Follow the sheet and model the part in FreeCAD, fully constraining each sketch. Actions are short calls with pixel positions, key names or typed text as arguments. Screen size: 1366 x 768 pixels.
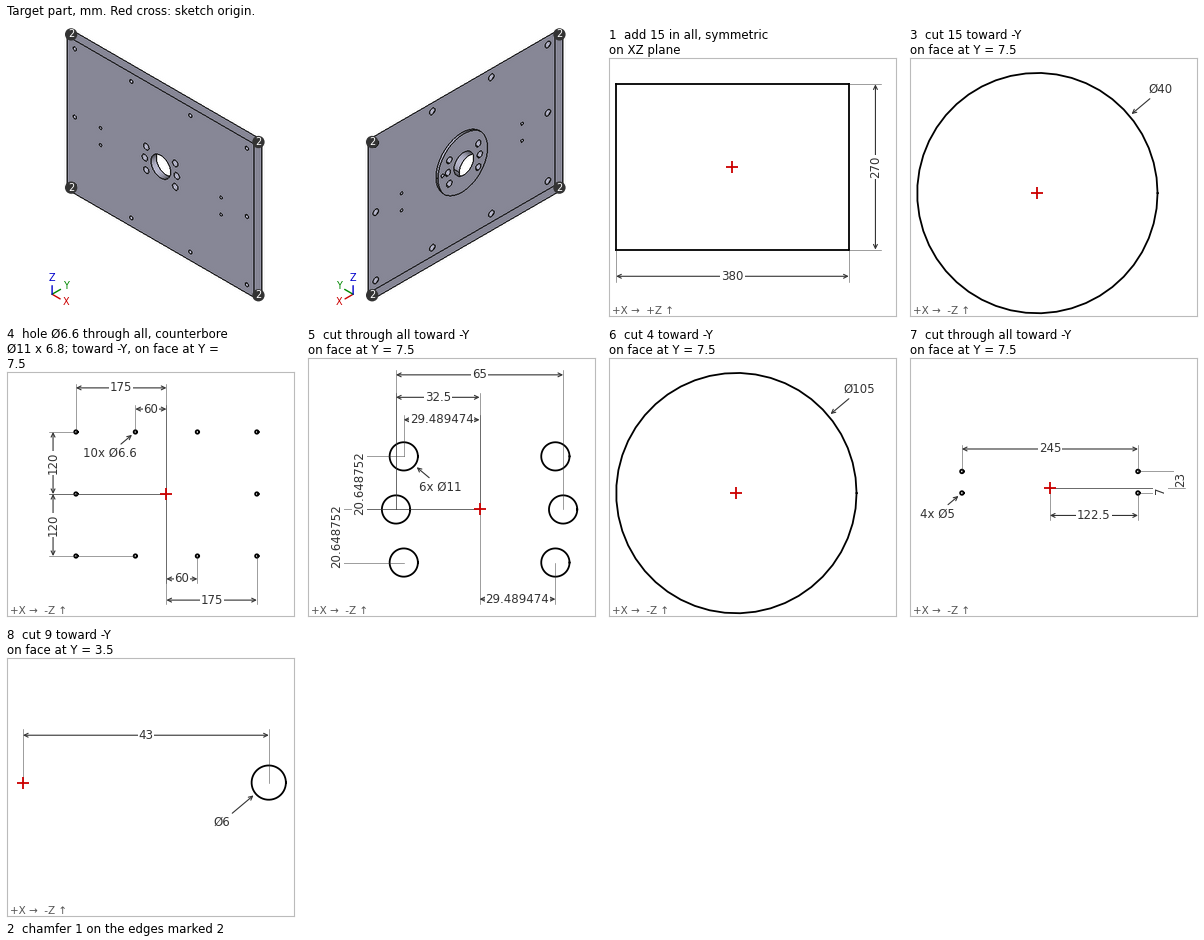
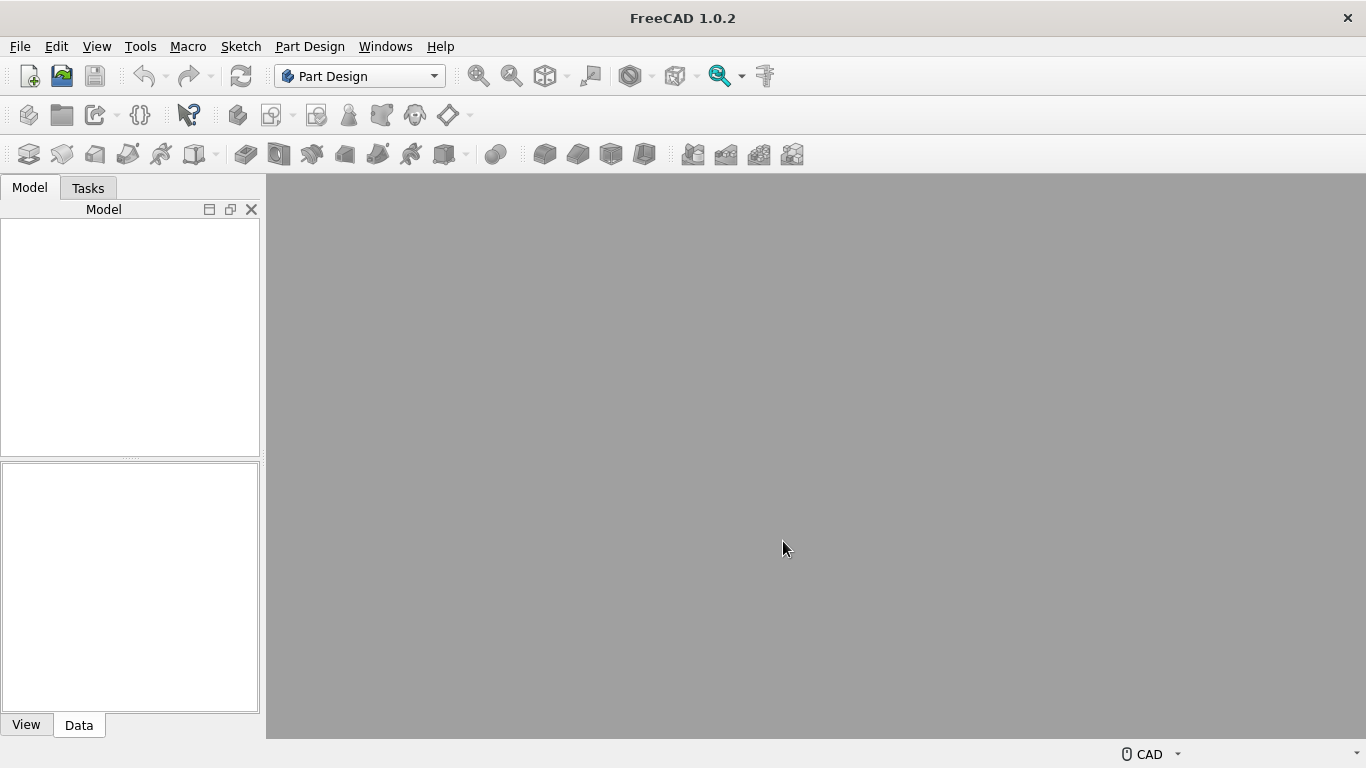
click(29, 76)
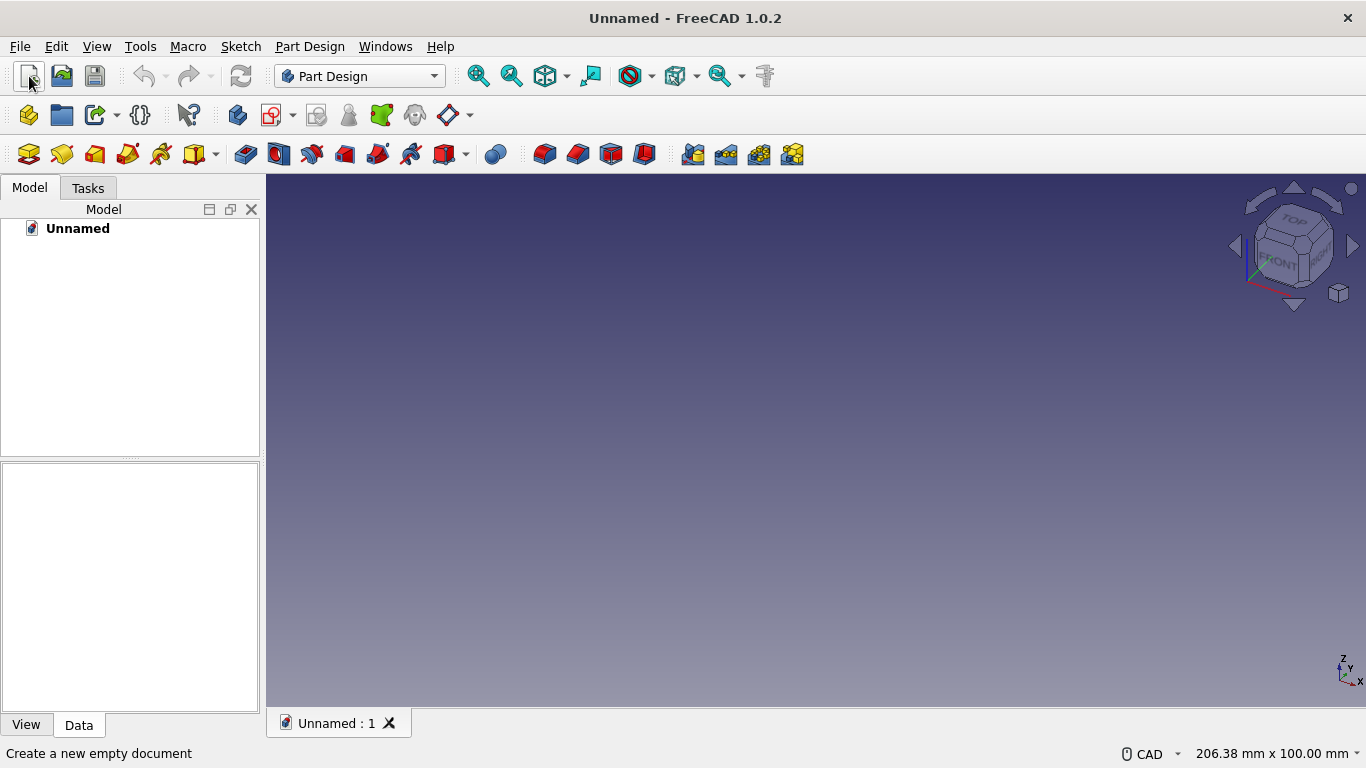
click(270, 116)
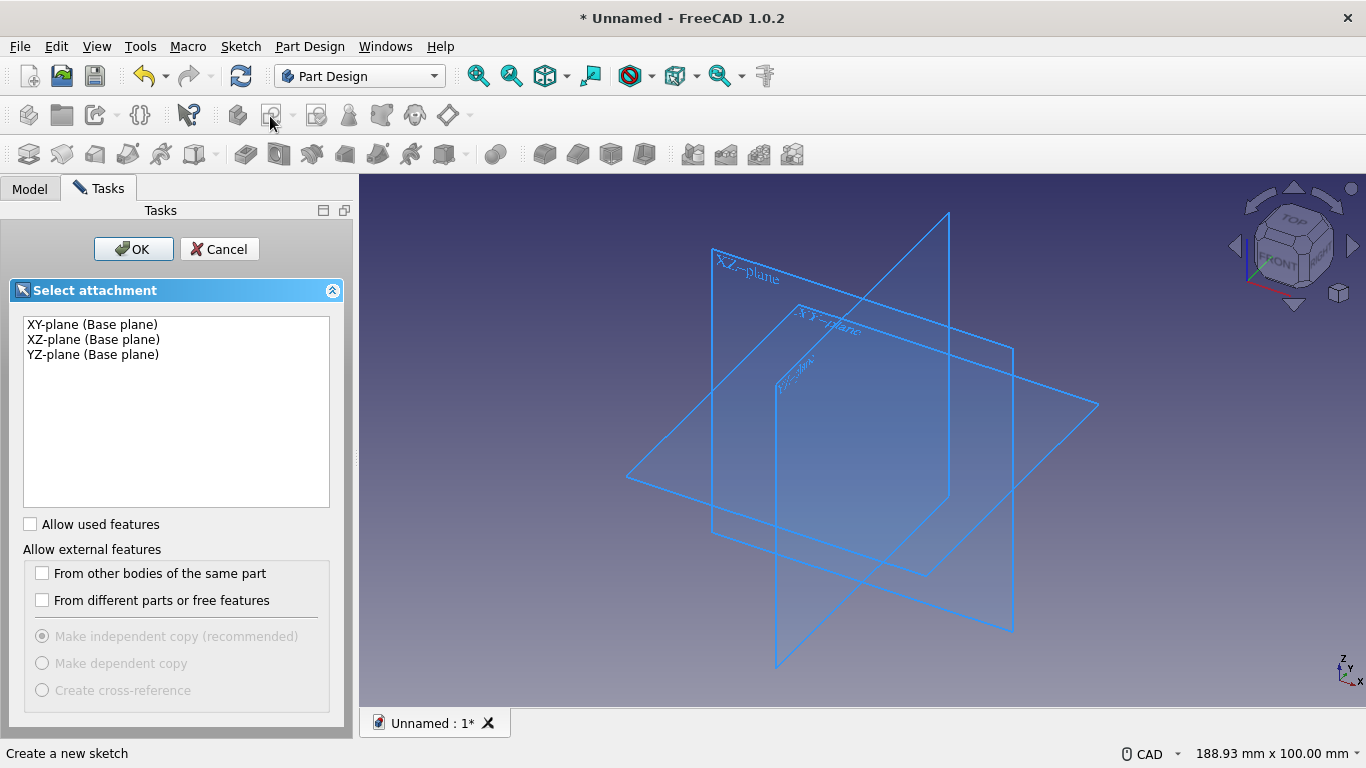
click(84, 340)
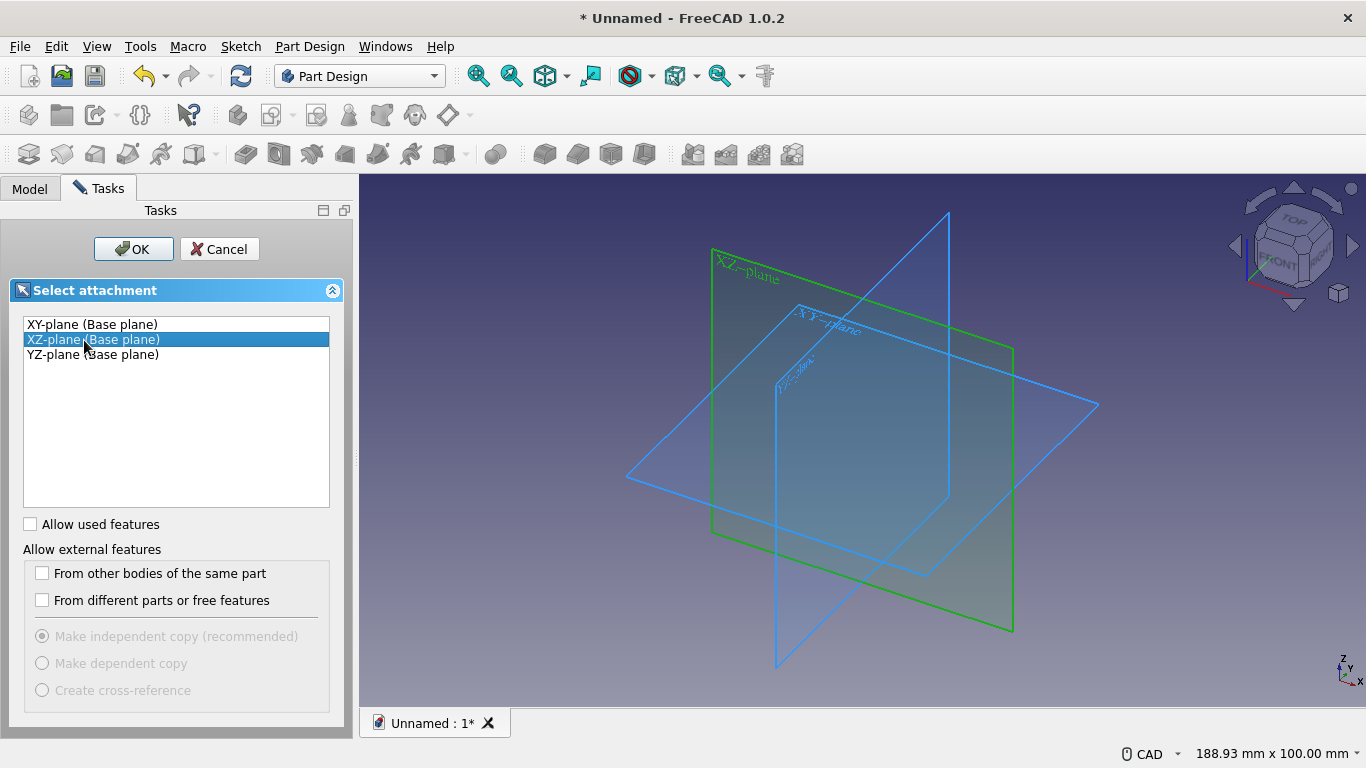
click(134, 249)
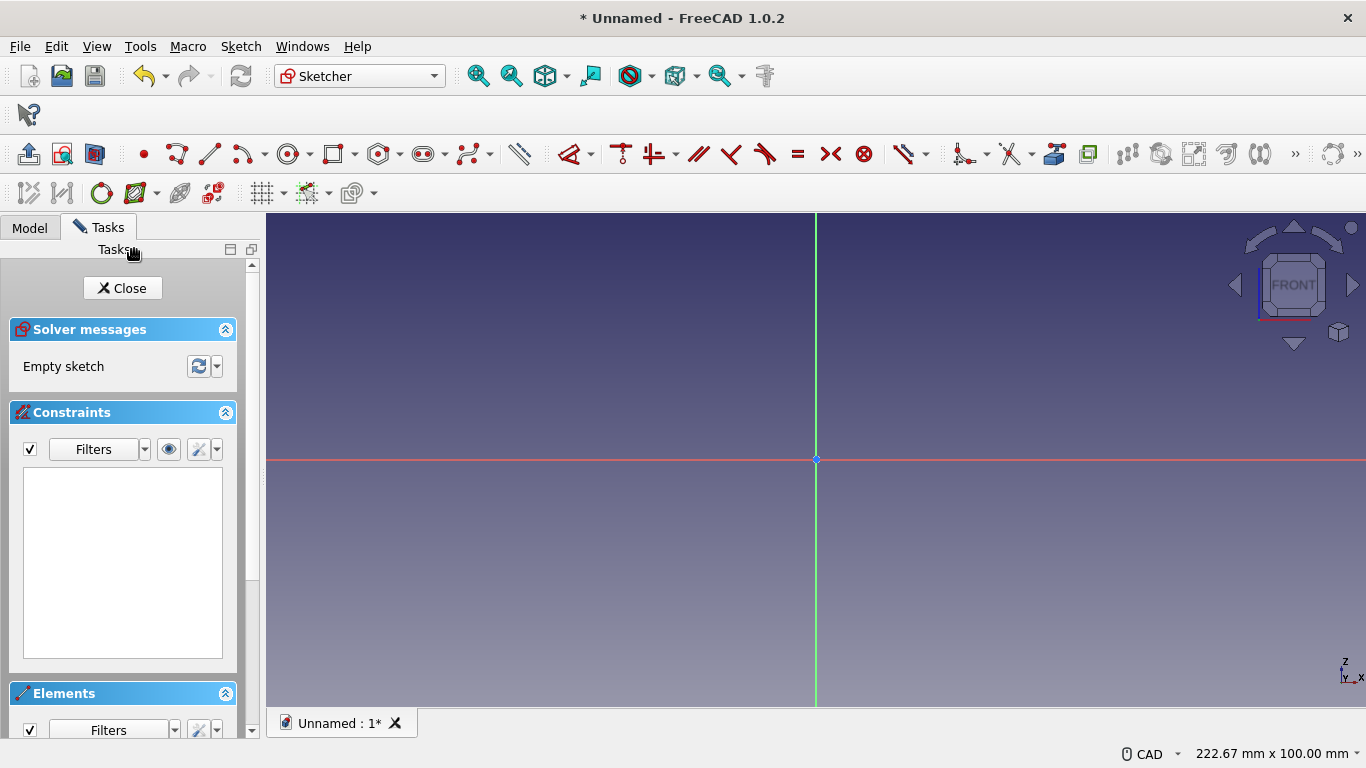
scroll(725, 460, down, 7)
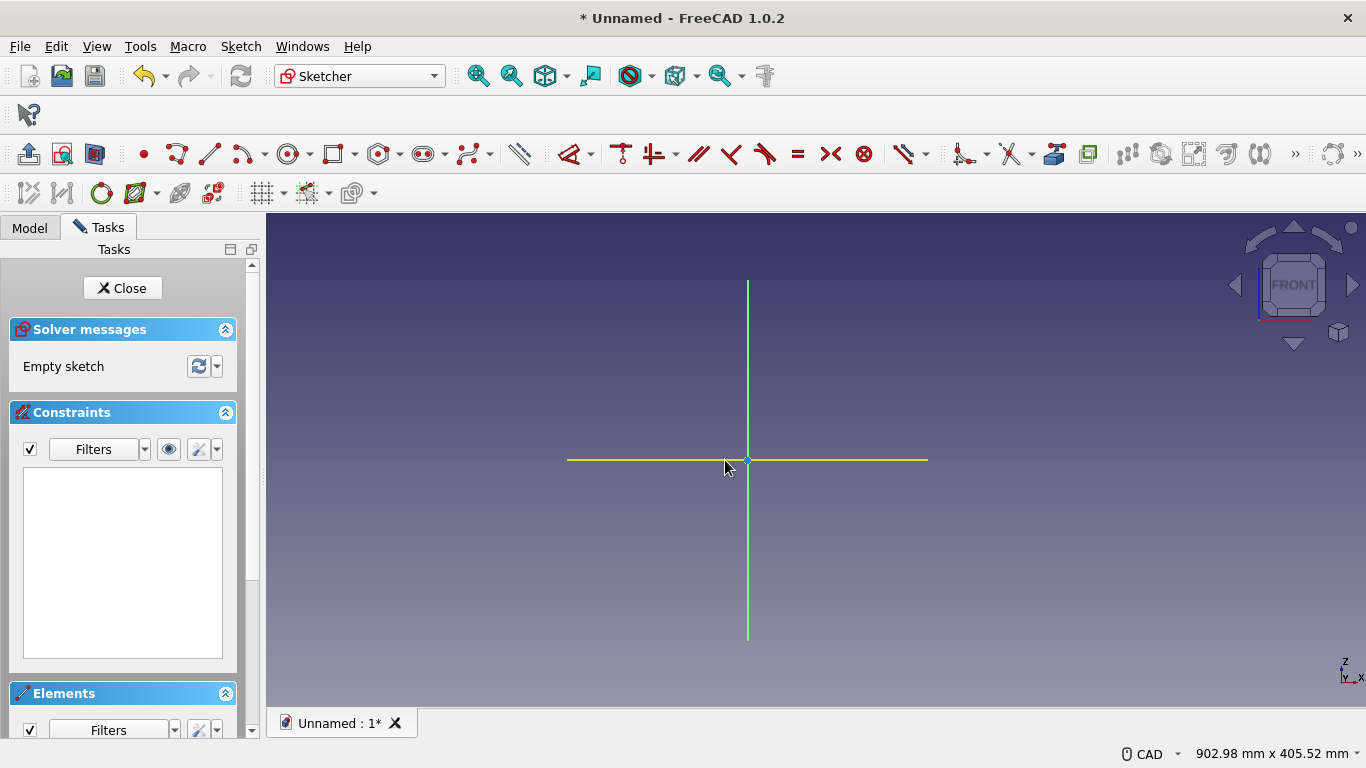
click(354, 154)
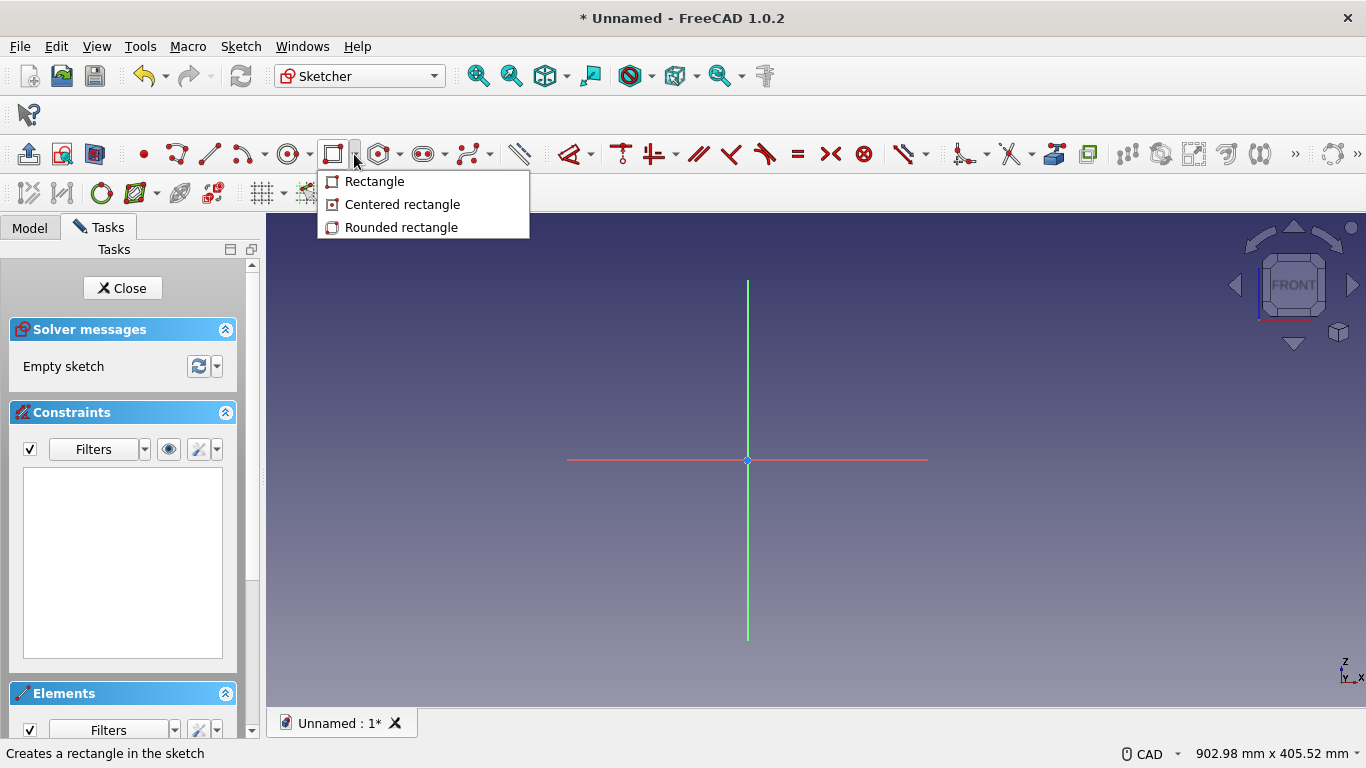
click(424, 204)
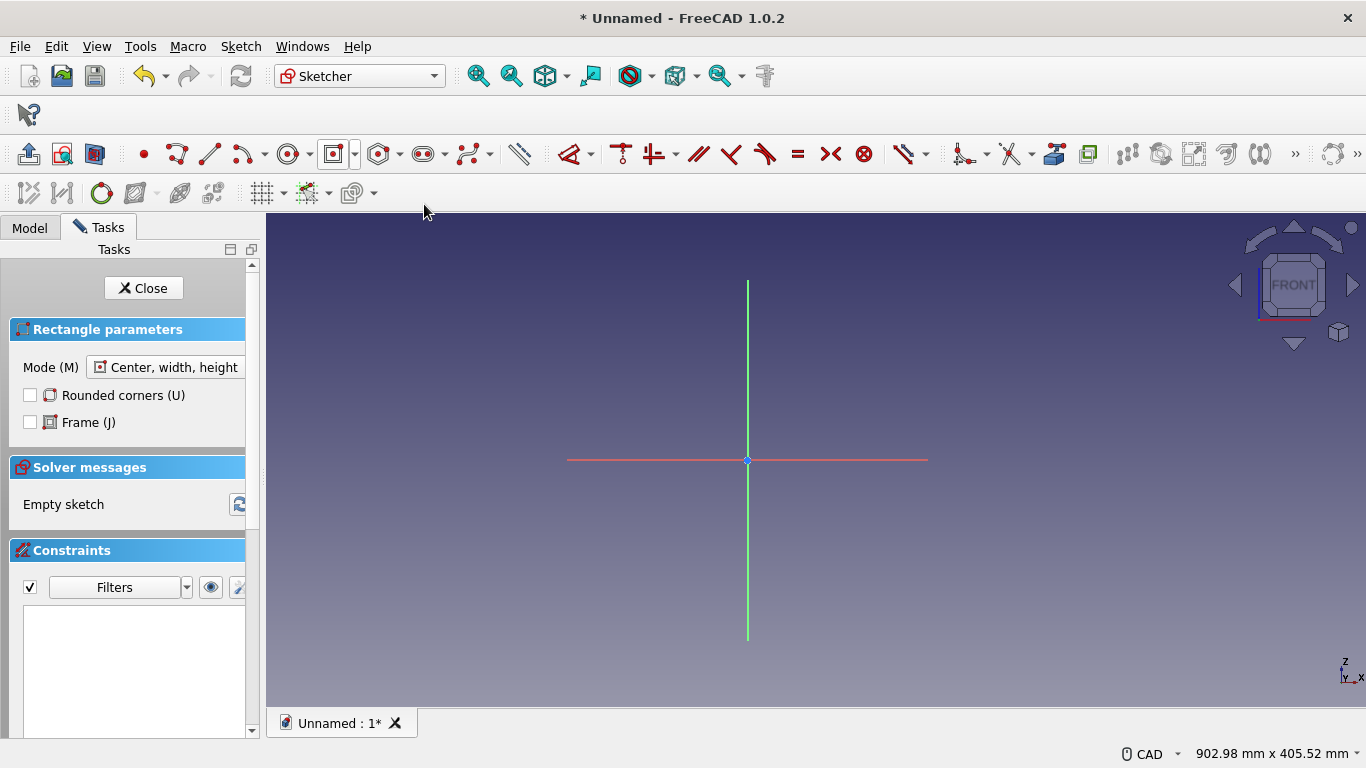
click(748, 460)
click(979, 296)
key(Escape)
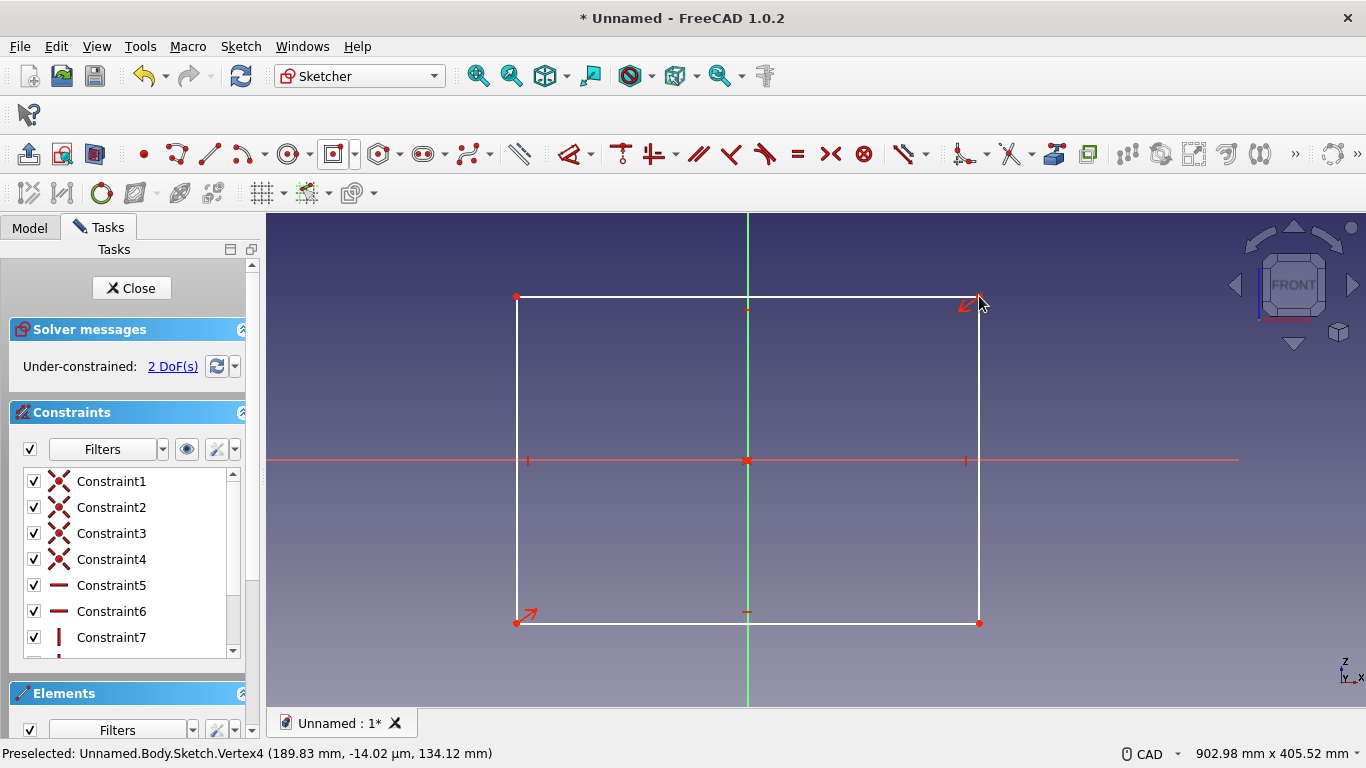
click(568, 154)